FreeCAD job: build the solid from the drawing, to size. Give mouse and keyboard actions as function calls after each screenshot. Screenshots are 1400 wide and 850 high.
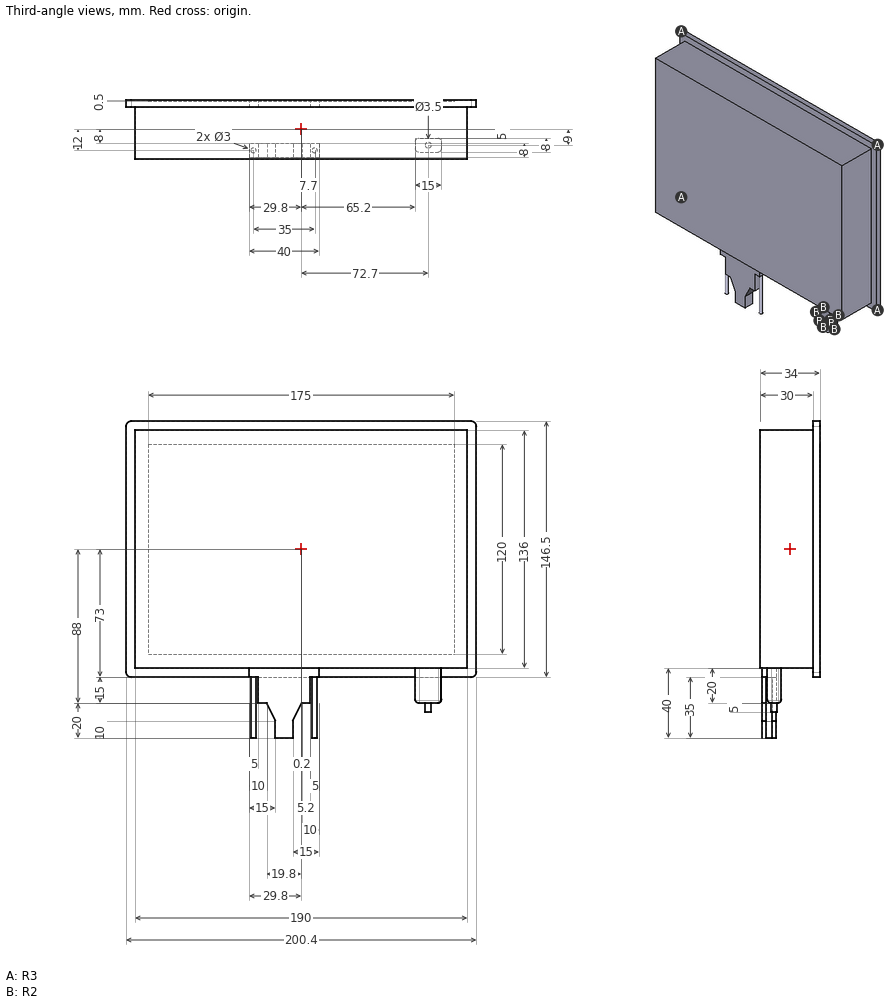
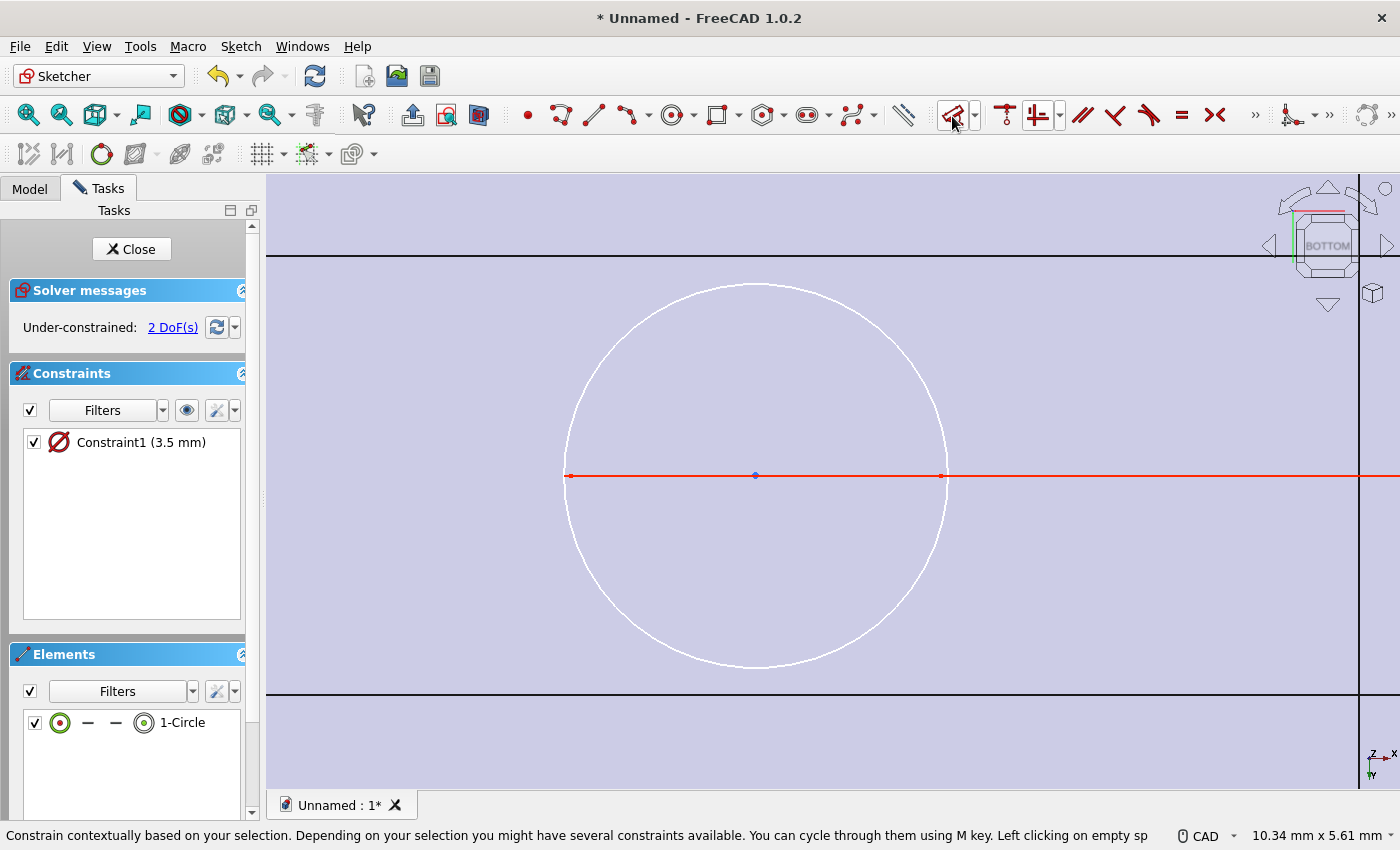
click(756, 476)
click(790, 618)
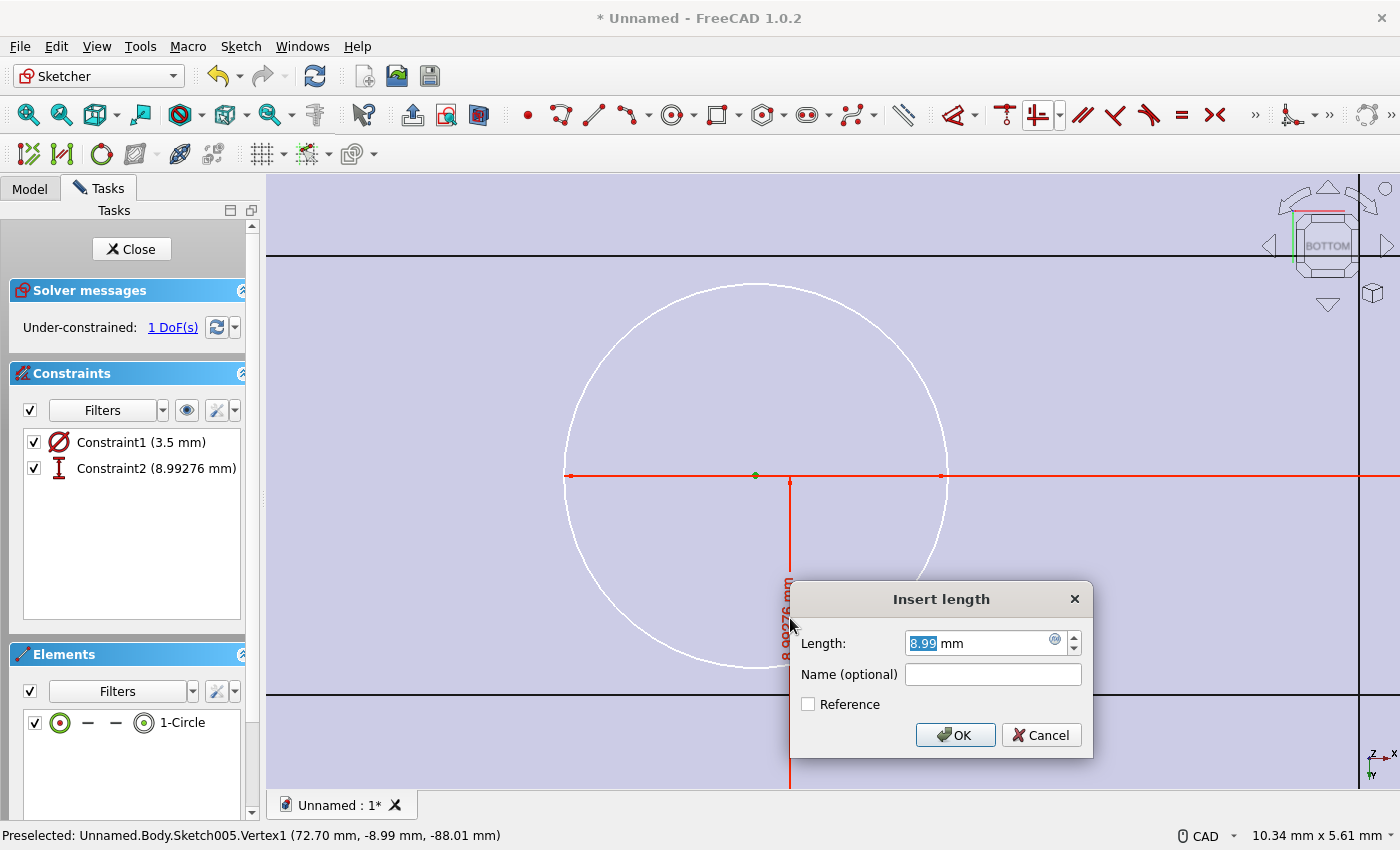
text(9)
key(Return)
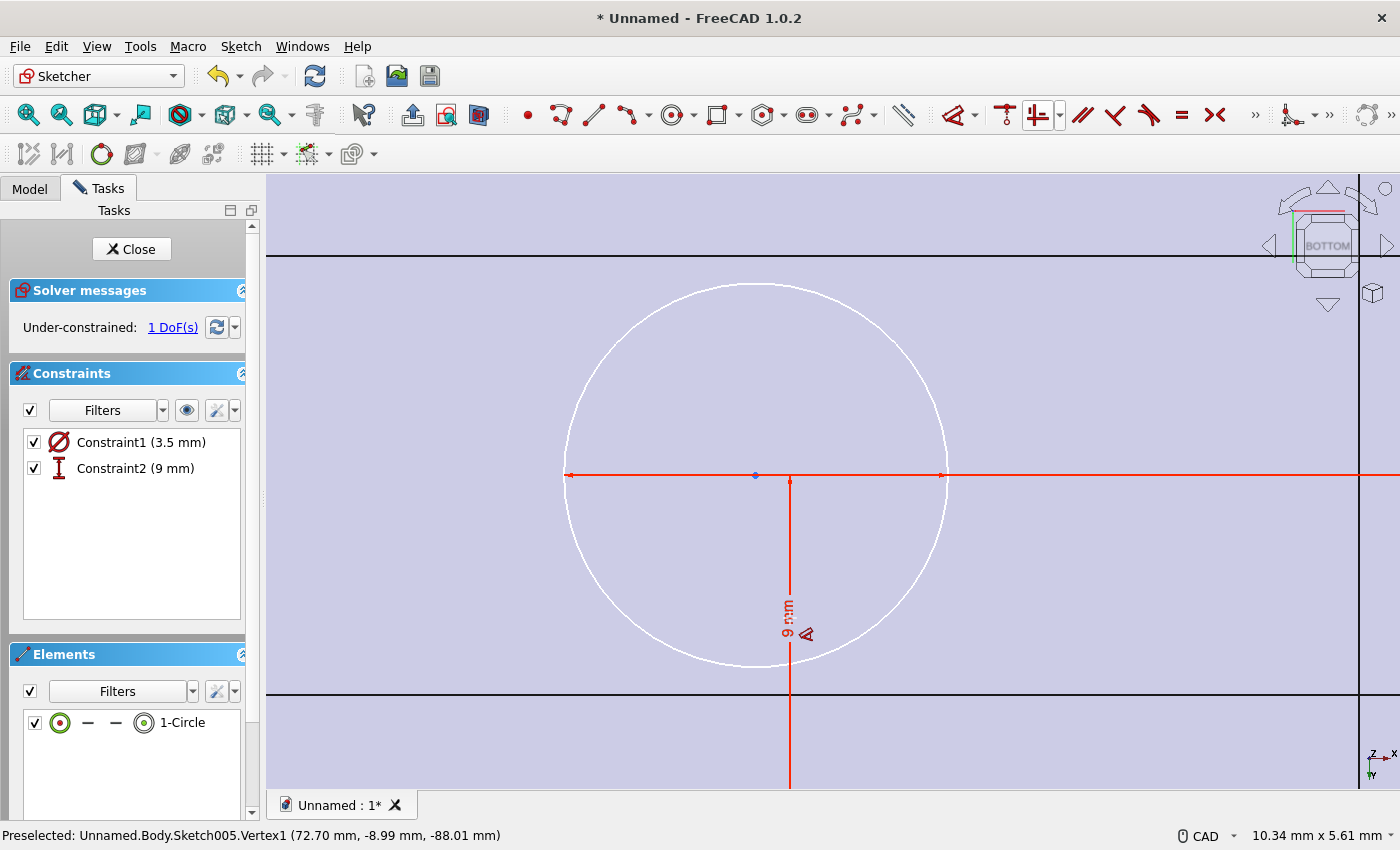
click(756, 475)
click(525, 441)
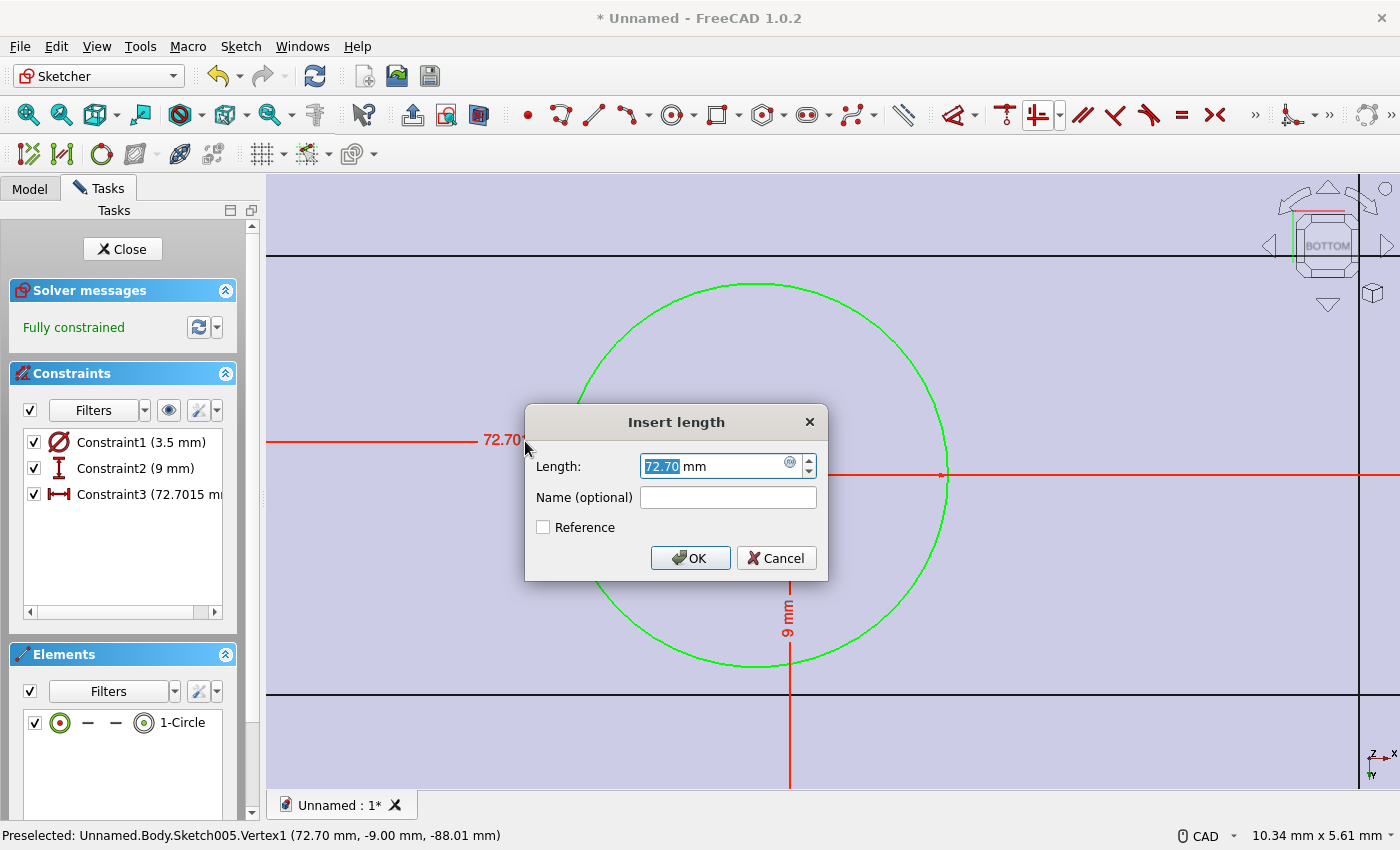
text(72.7)
key(Return)
key(Escape)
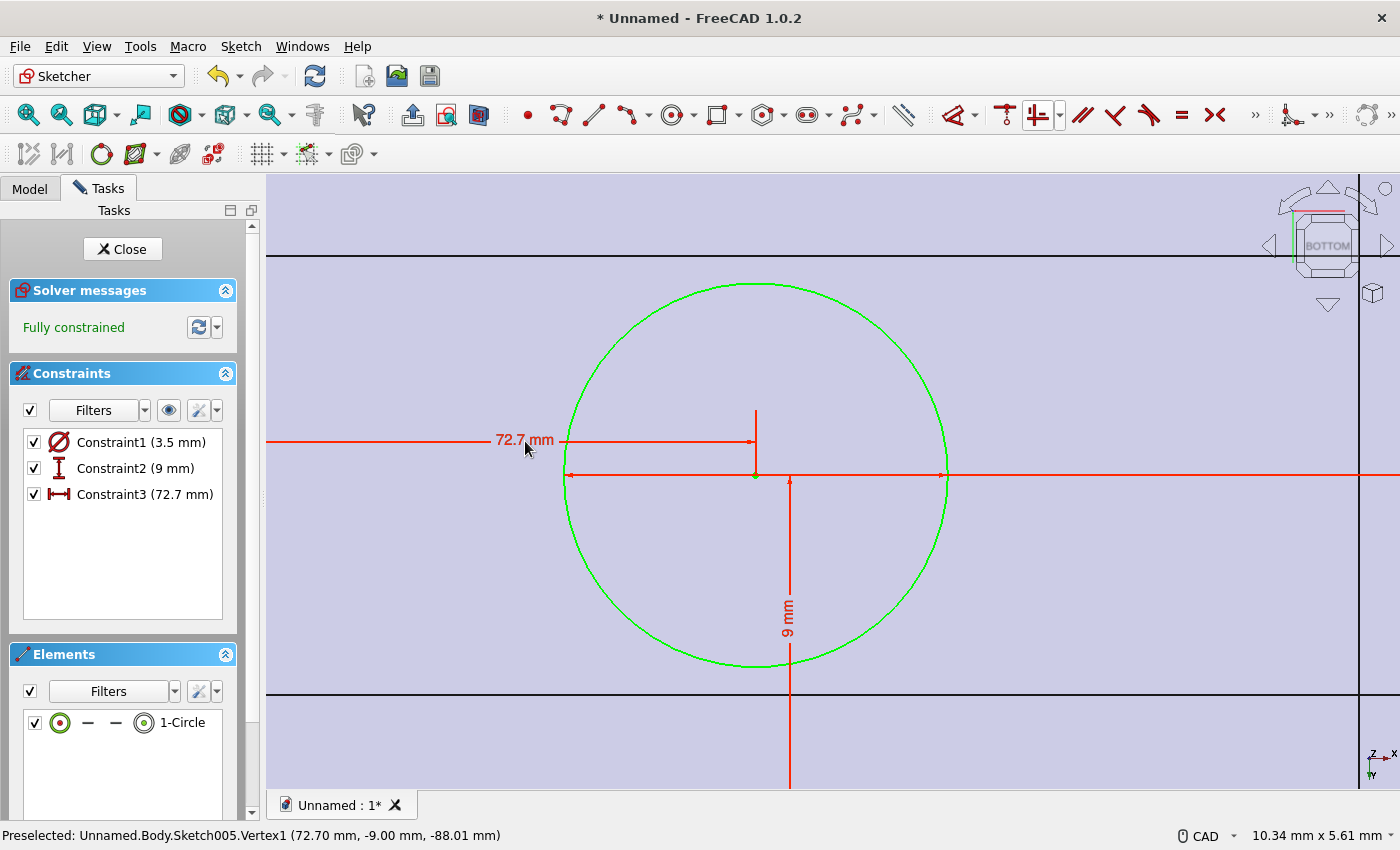
click(123, 249)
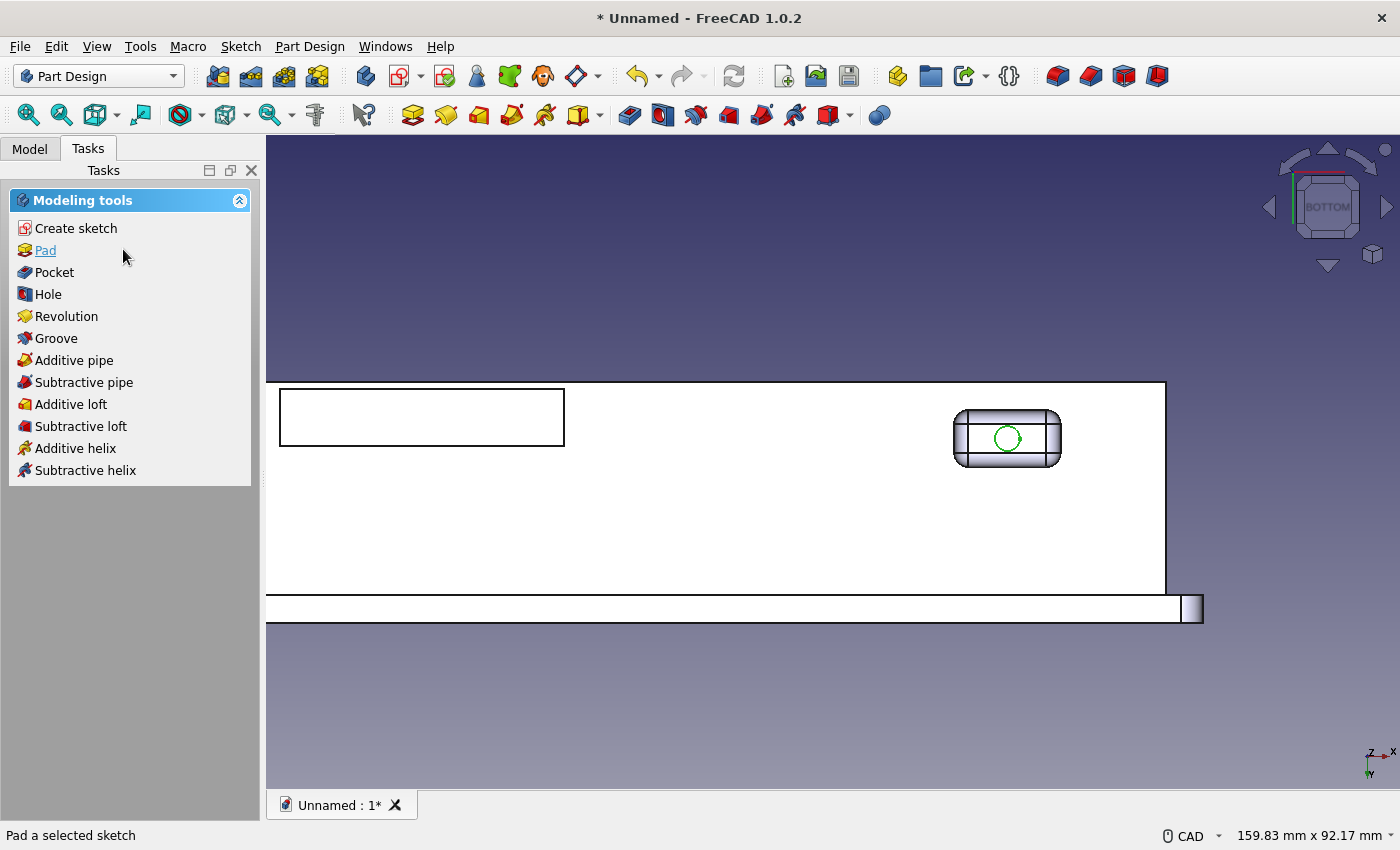
click(413, 116)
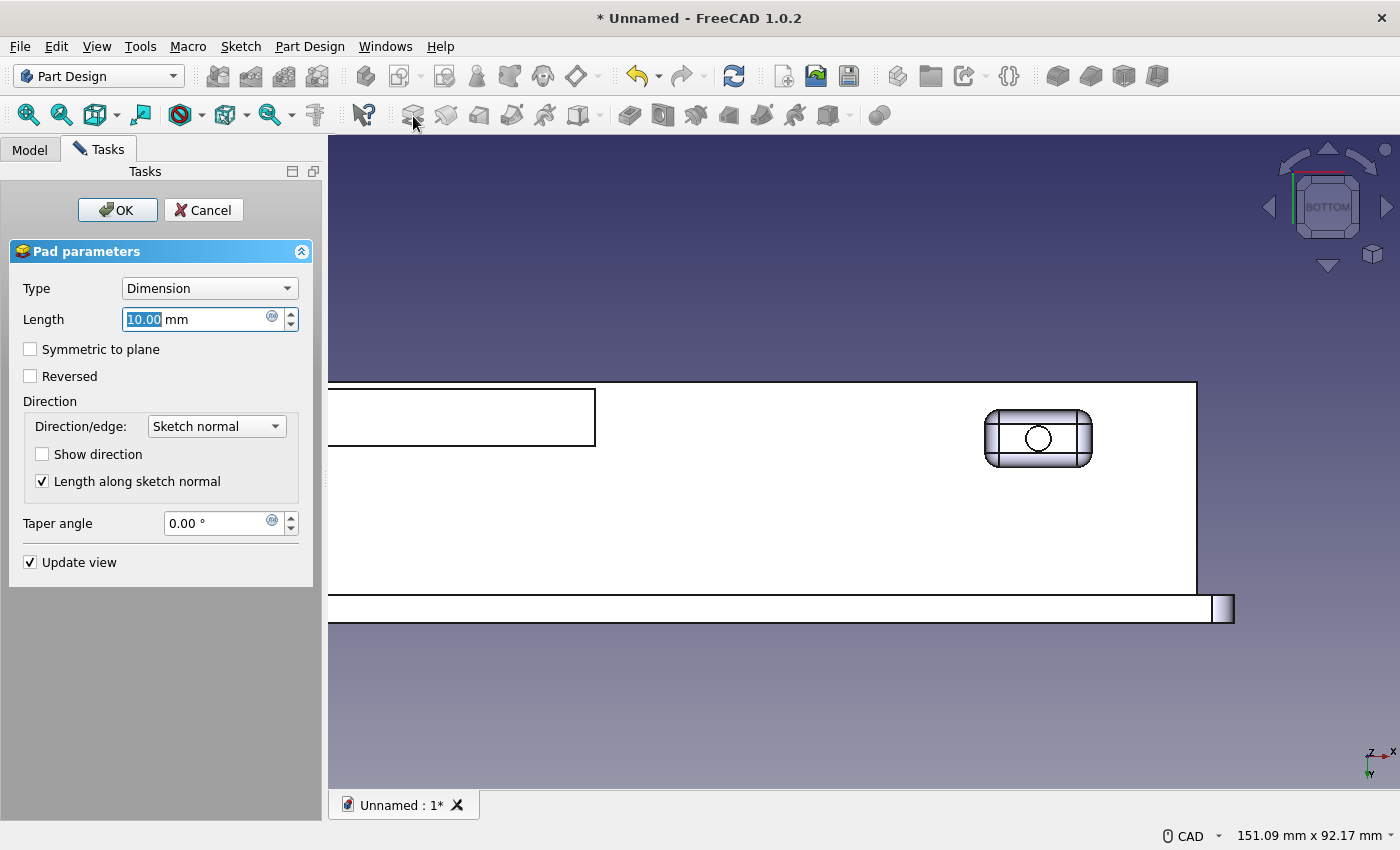
text(5)
key(Tab)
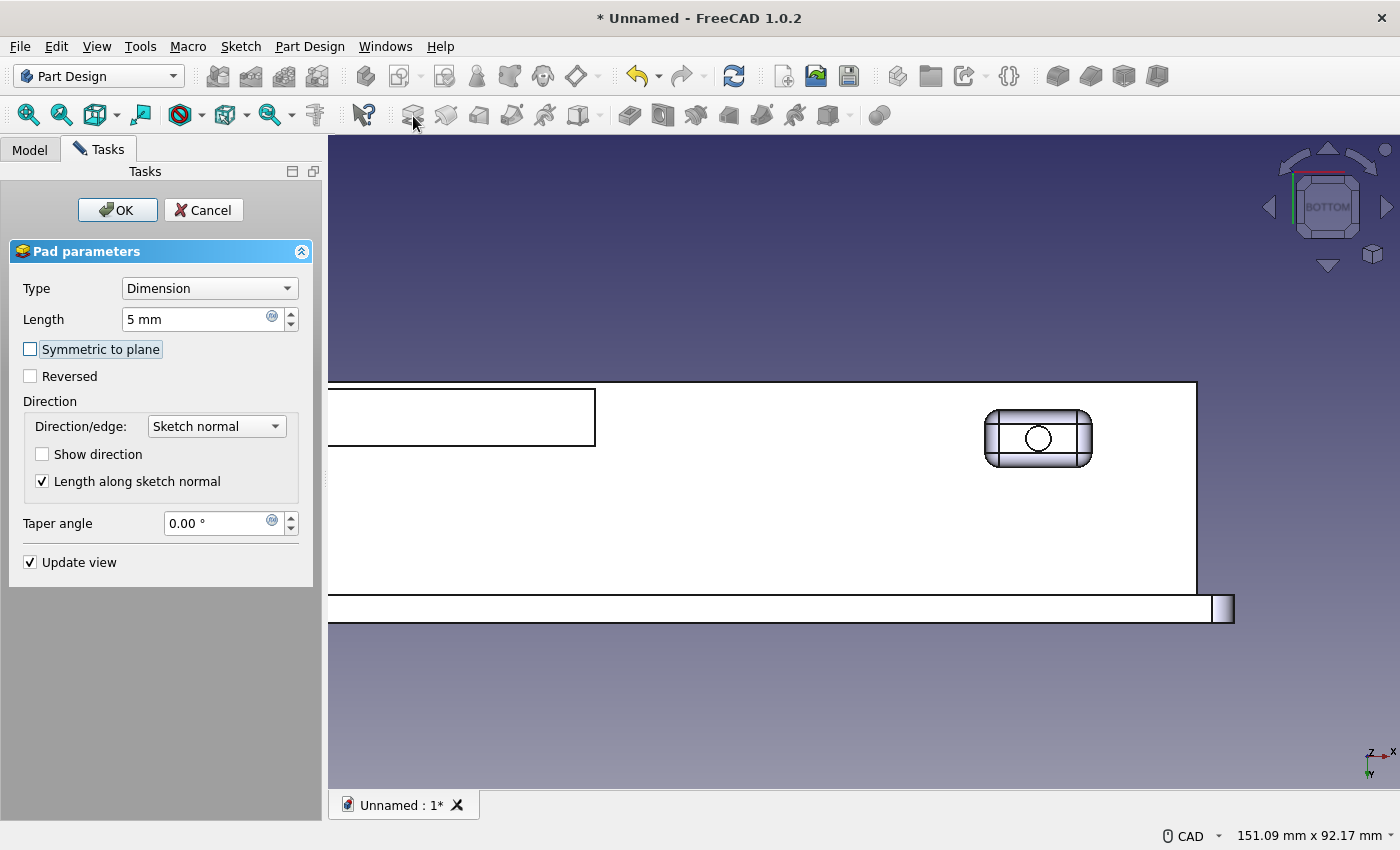
click(118, 210)